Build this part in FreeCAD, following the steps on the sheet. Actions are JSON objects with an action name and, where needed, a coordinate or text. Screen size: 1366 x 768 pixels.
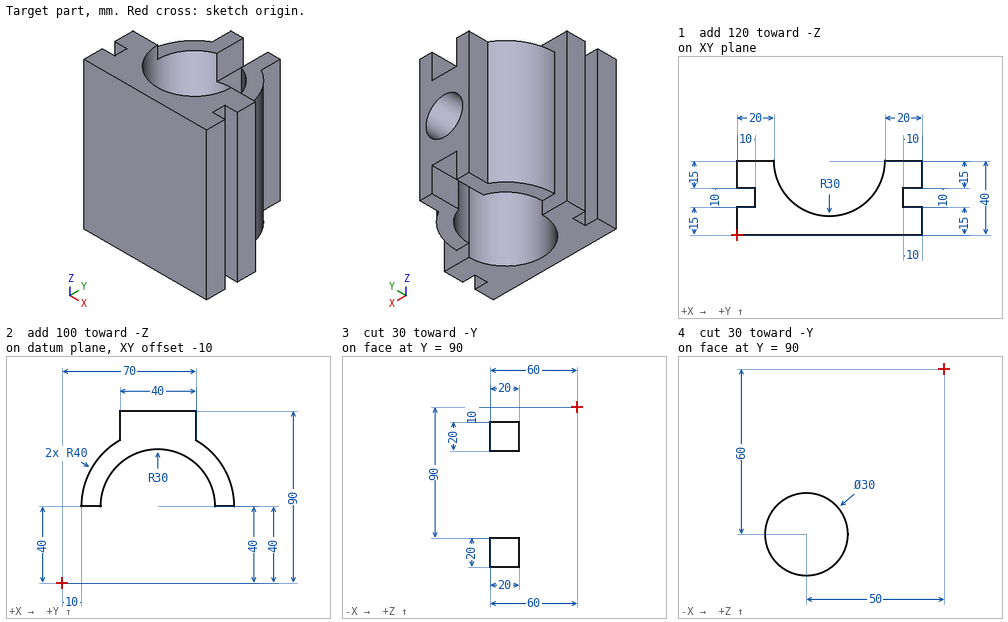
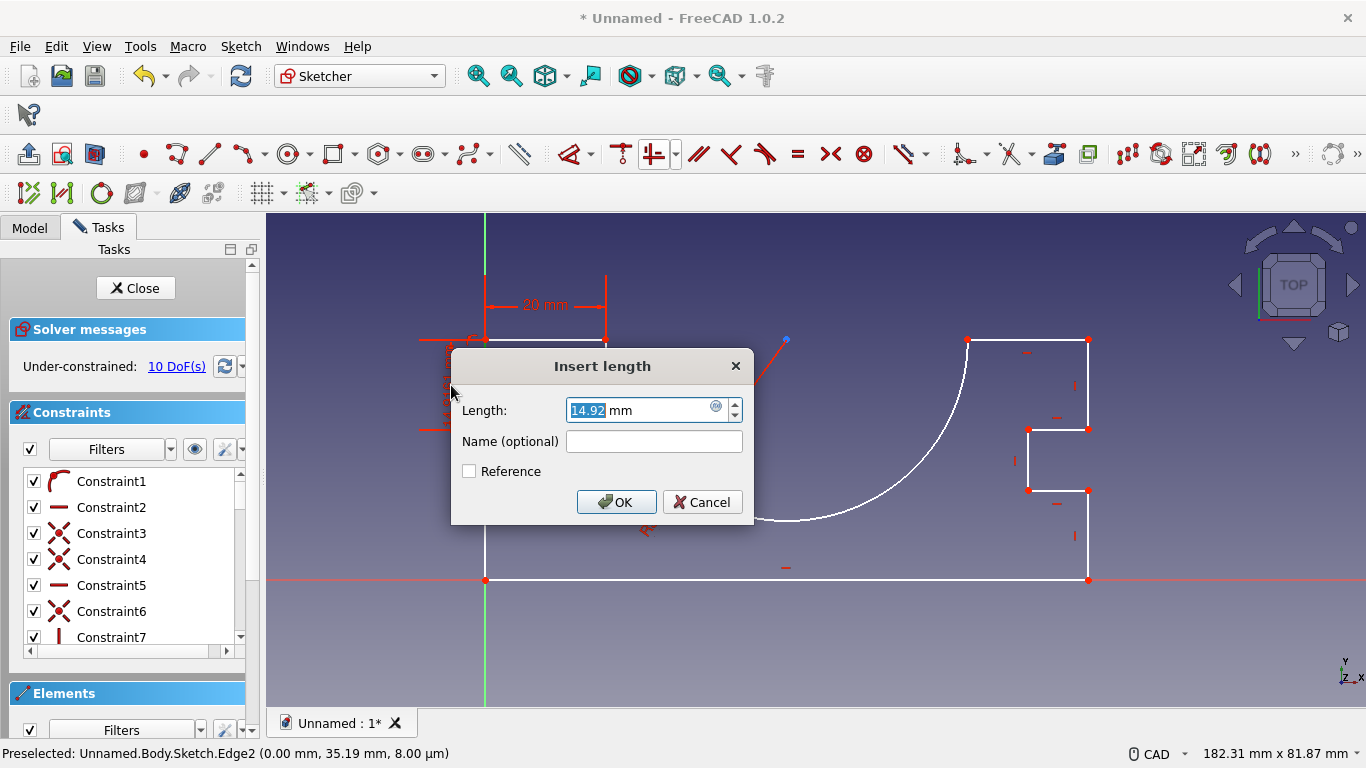
{"action": "type", "text": "15"}
{"action": "key", "text": "Return"}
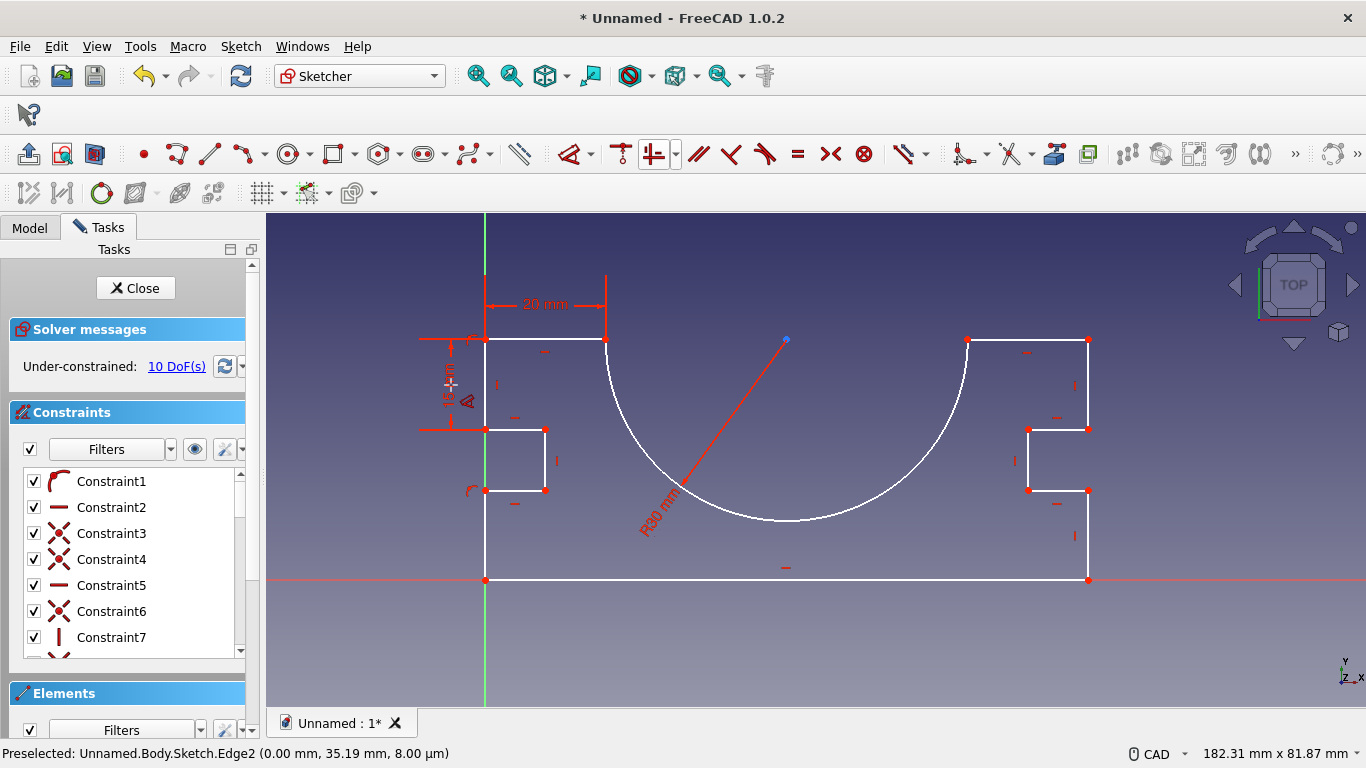
{"action": "left_click", "coordinate": [503, 430]}
{"action": "left_click", "coordinate": [529, 396]}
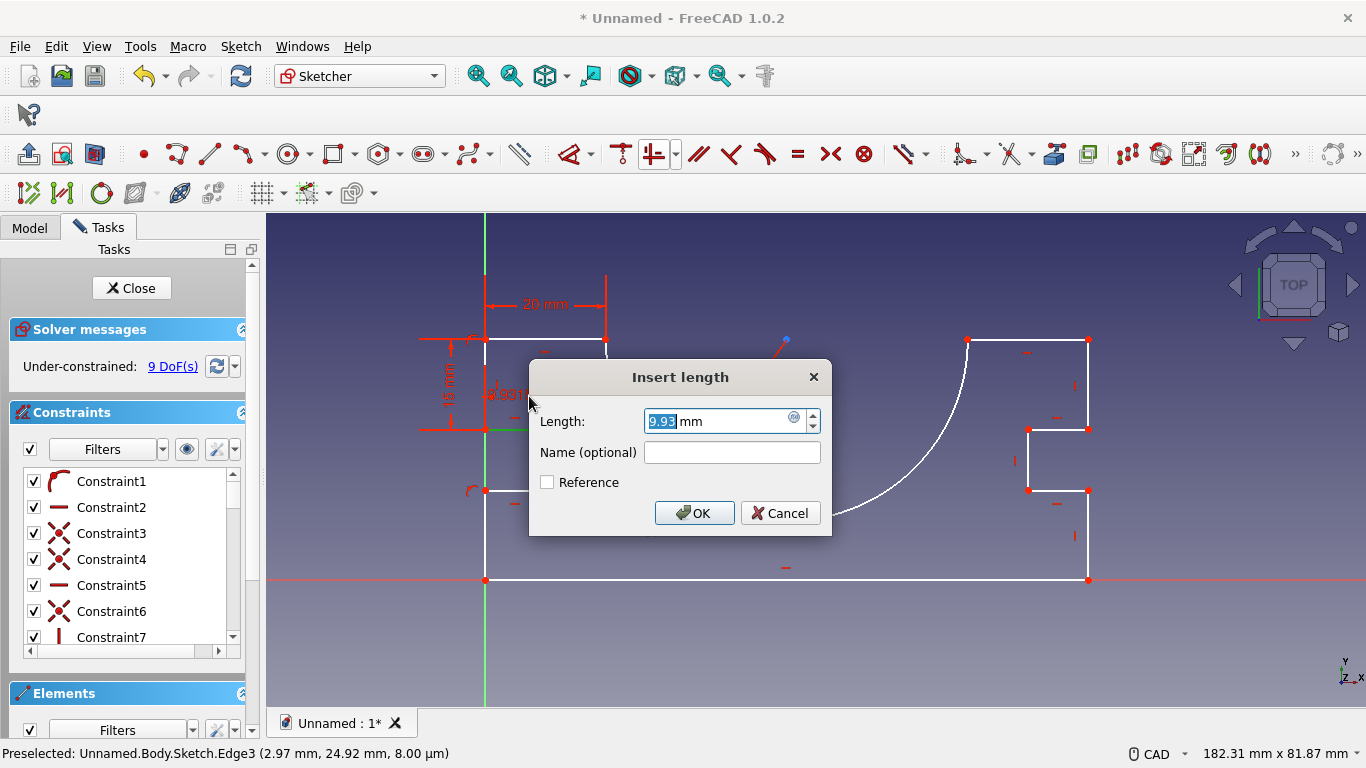
{"action": "type", "text": "10"}
{"action": "key", "text": "Return"}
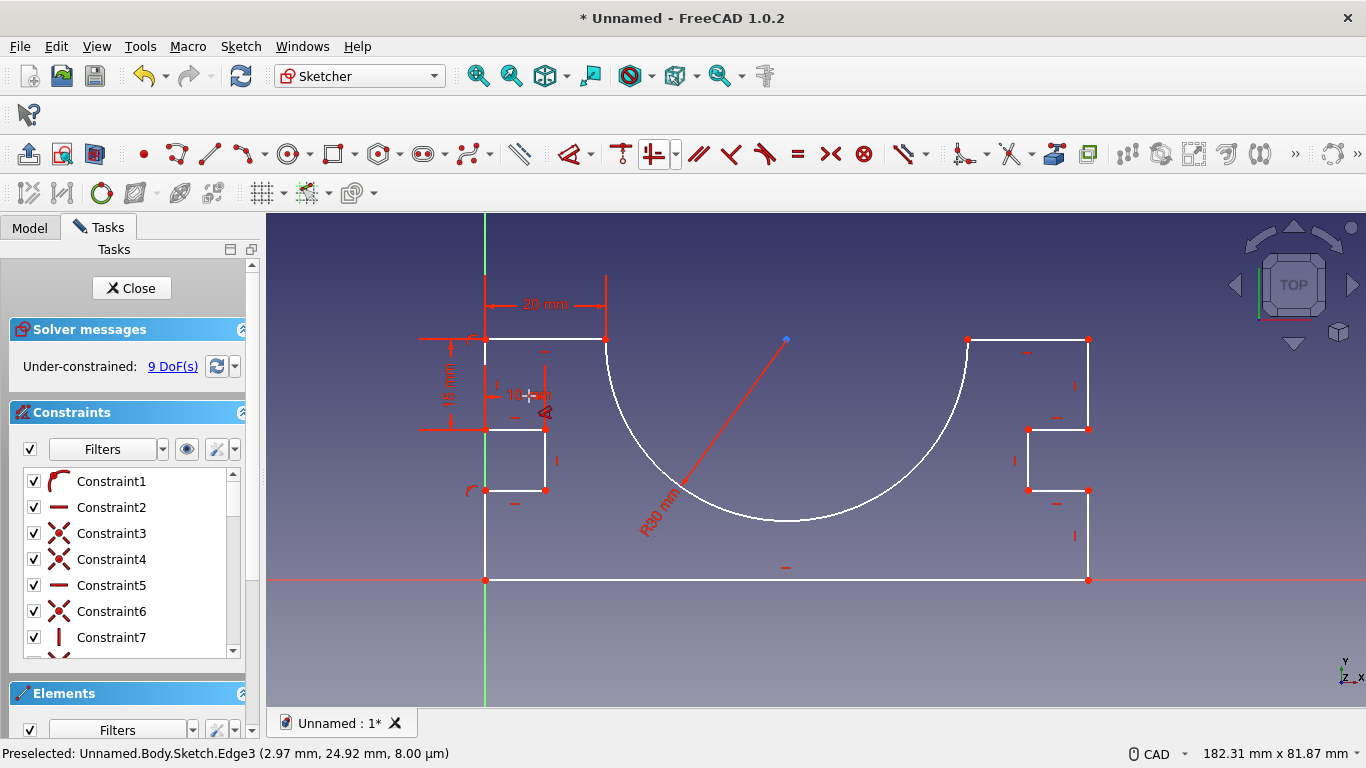
{"action": "left_click", "coordinate": [545, 448]}
{"action": "left_click", "coordinate": [511, 460]}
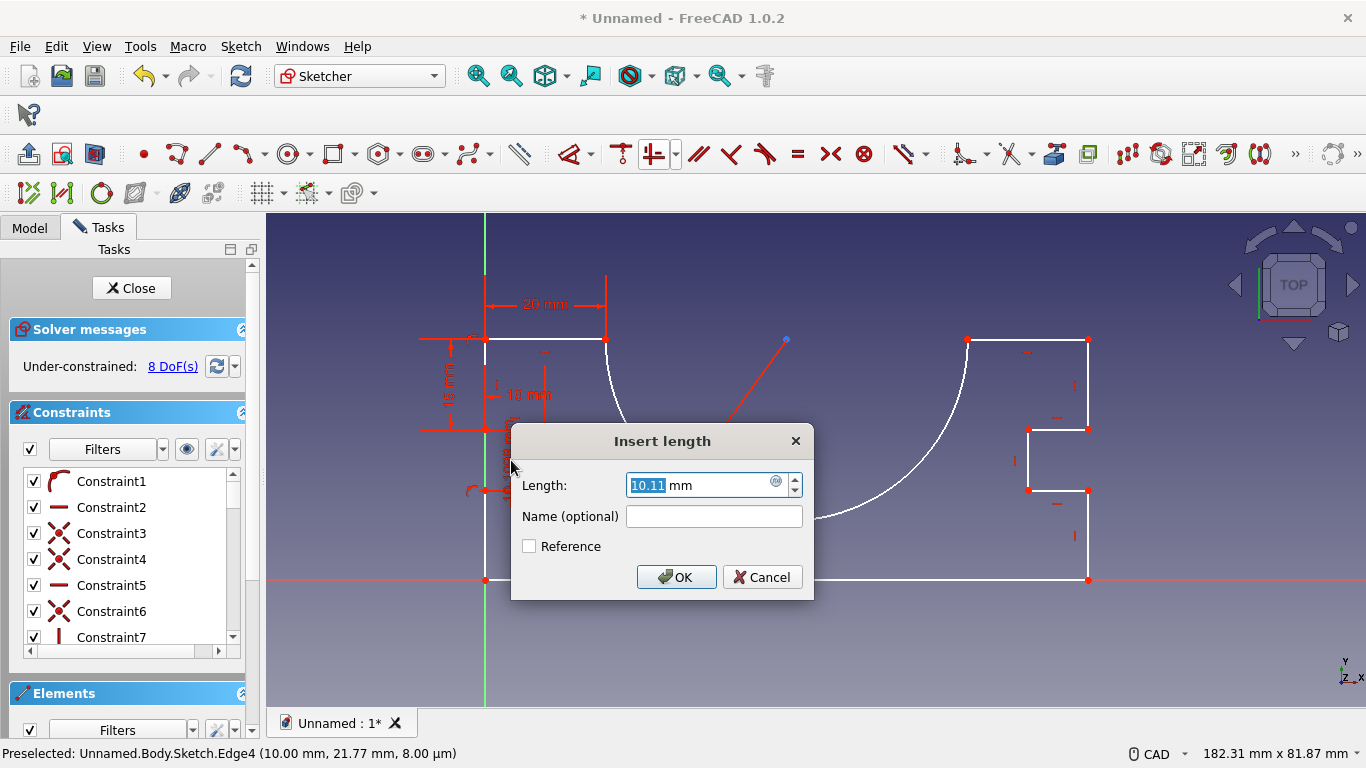
{"action": "type", "text": "10"}
{"action": "key", "text": "Return"}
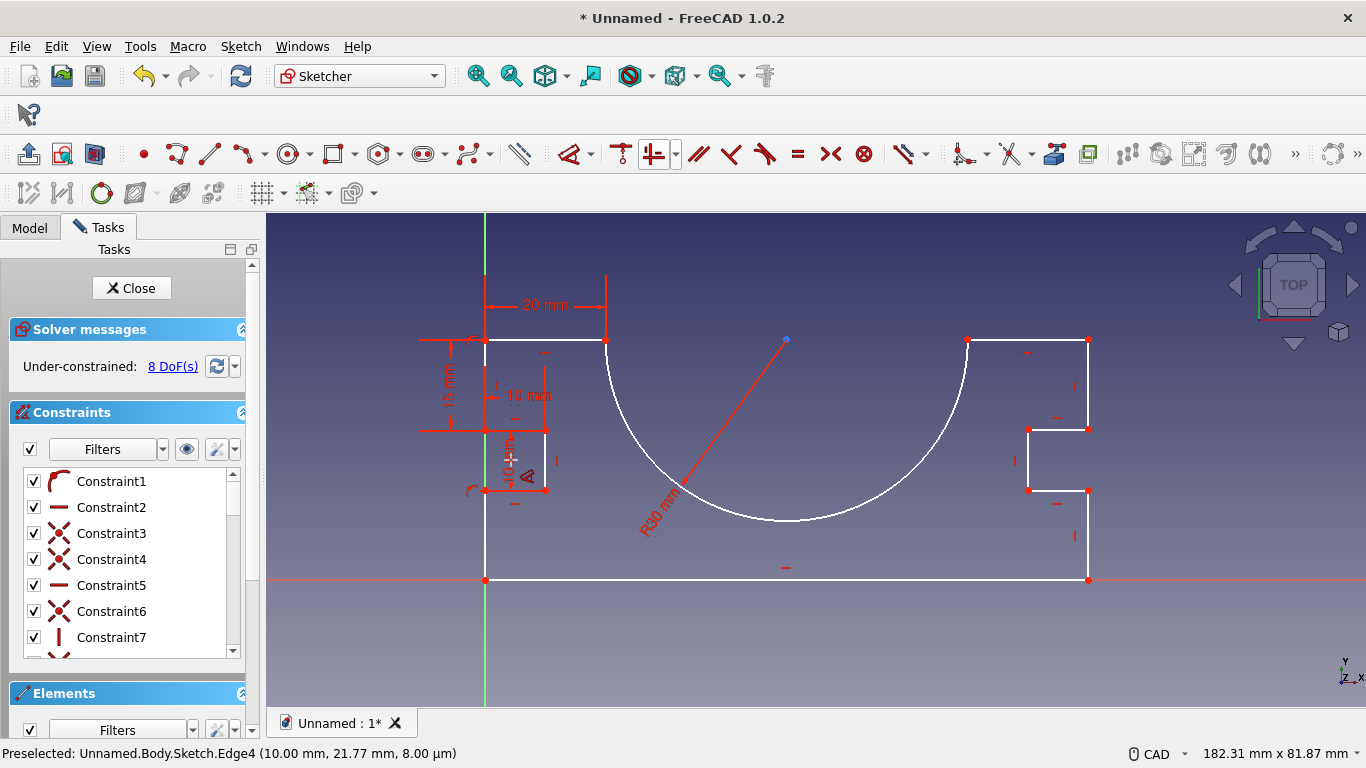
{"action": "left_click", "coordinate": [485, 518]}
{"action": "left_click", "coordinate": [451, 536]}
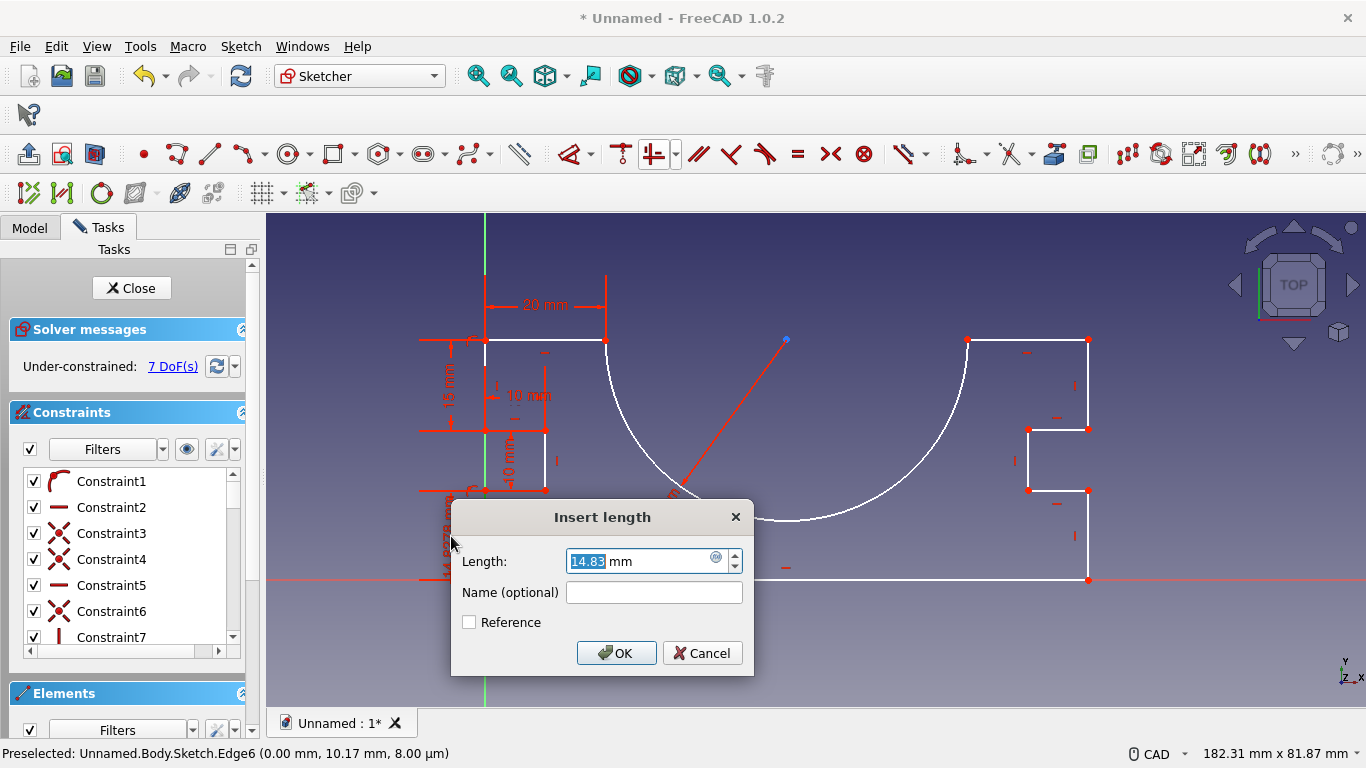
{"action": "type", "text": "15"}
{"action": "key", "text": "Return"}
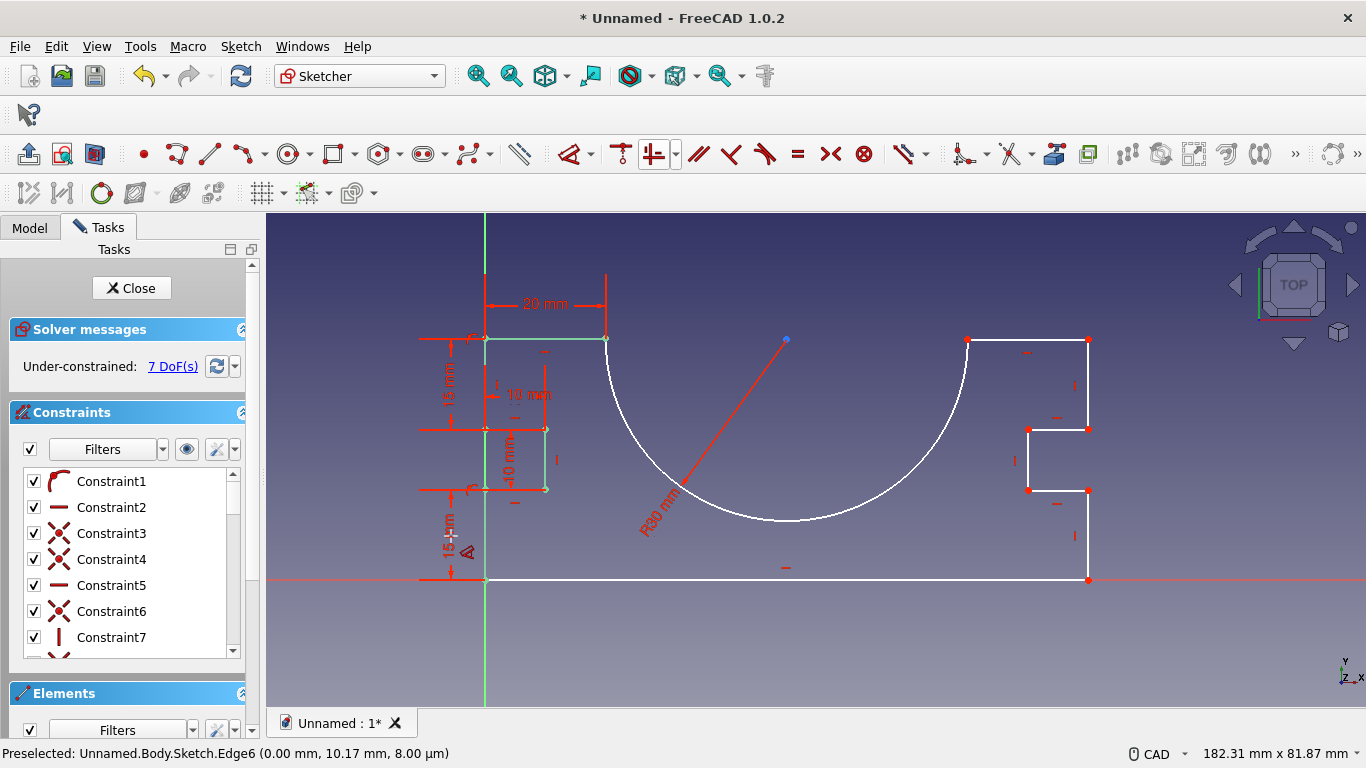
{"action": "left_click", "coordinate": [1088, 554]}
{"action": "left_click", "coordinate": [1122, 536]}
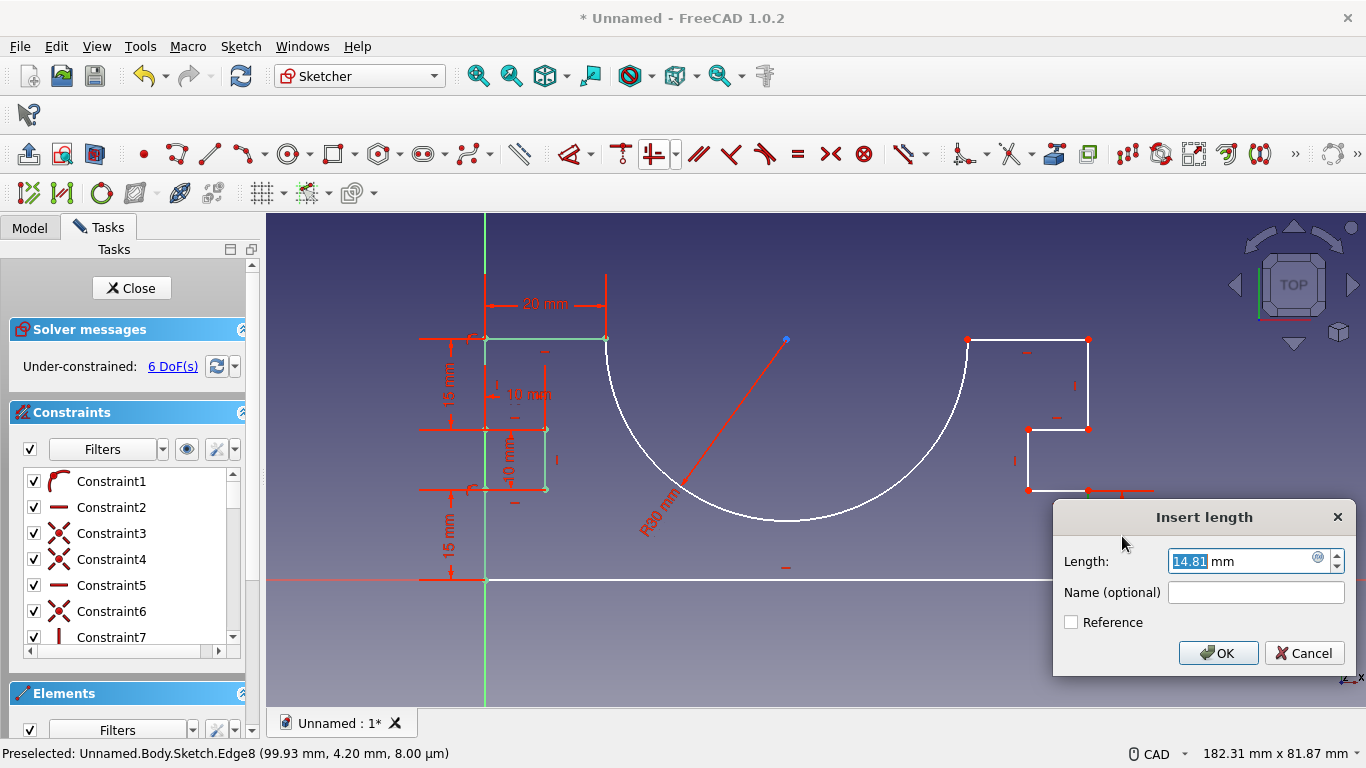
{"action": "type", "text": "15"}
{"action": "key", "text": "Return"}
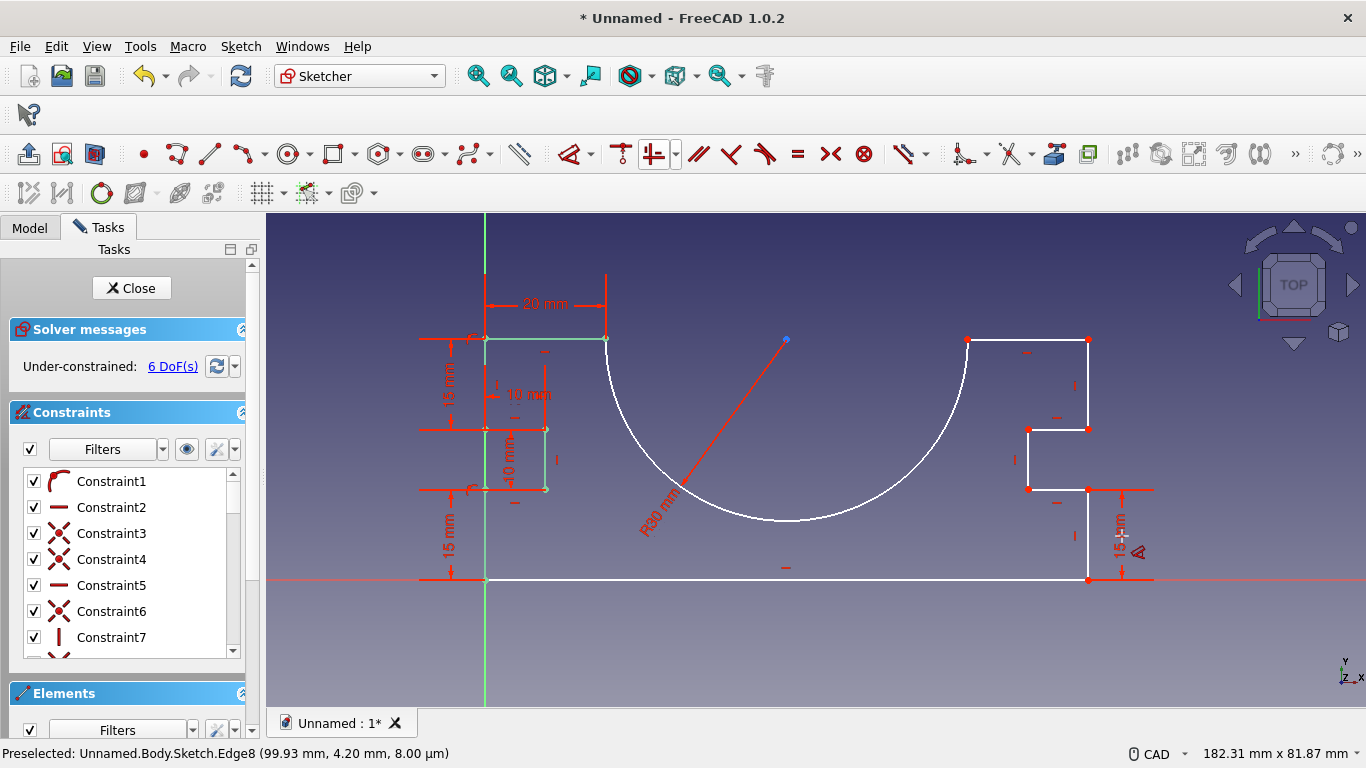
{"action": "left_click", "coordinate": [1070, 490]}
{"action": "left_click", "coordinate": [1044, 524]}